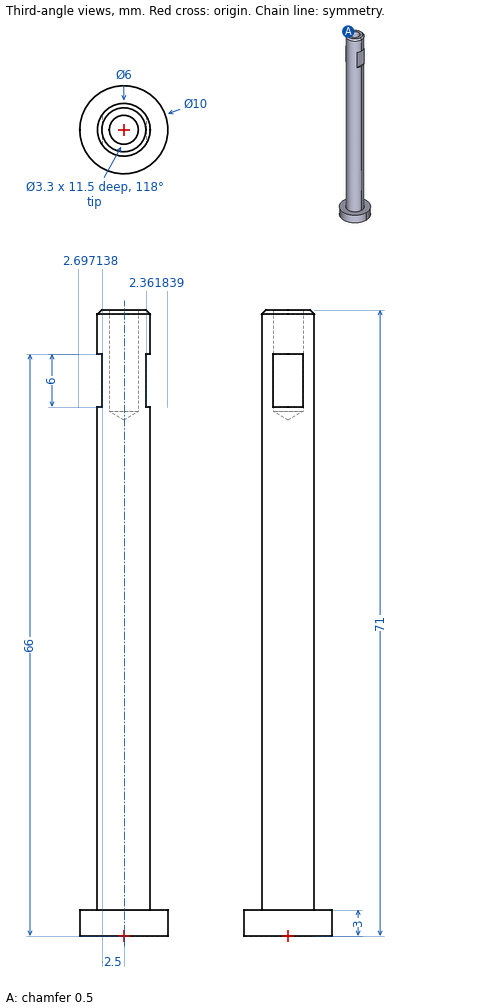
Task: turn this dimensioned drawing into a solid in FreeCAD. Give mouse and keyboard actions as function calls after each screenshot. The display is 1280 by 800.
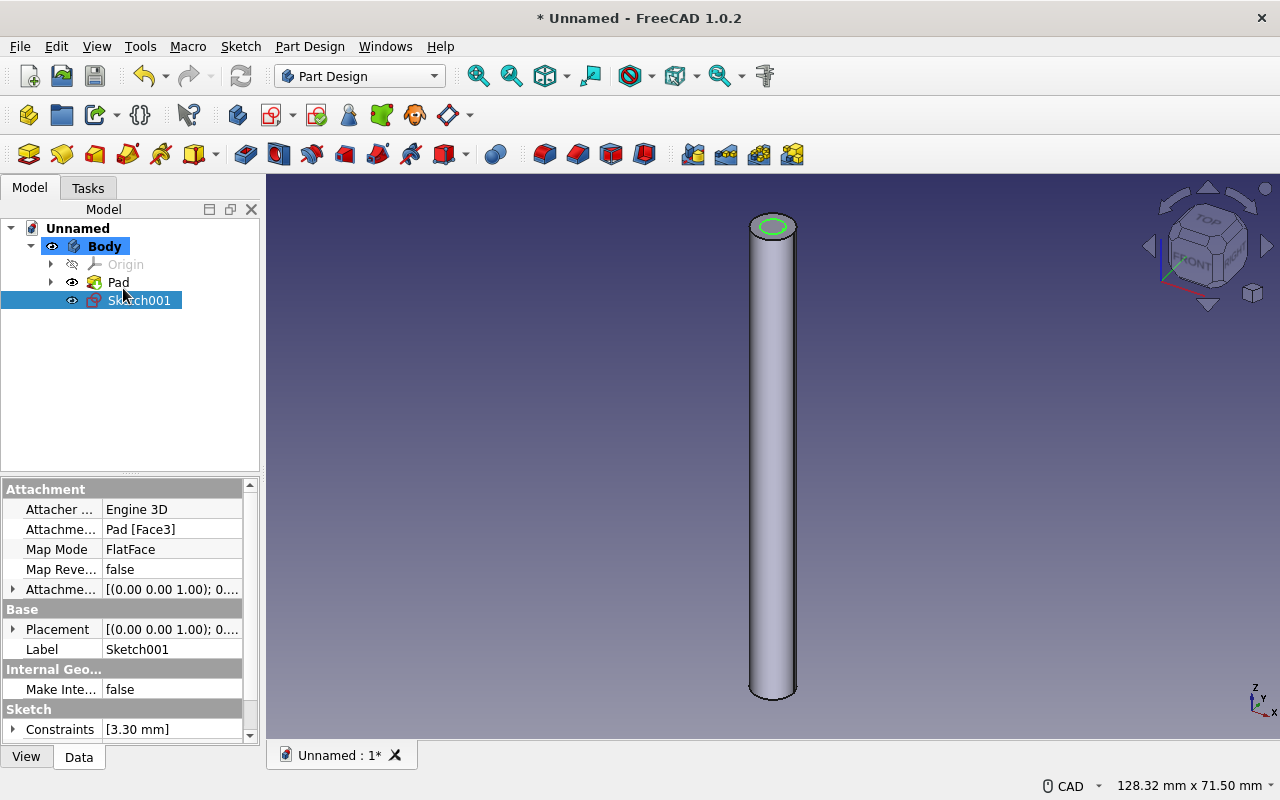
click(279, 154)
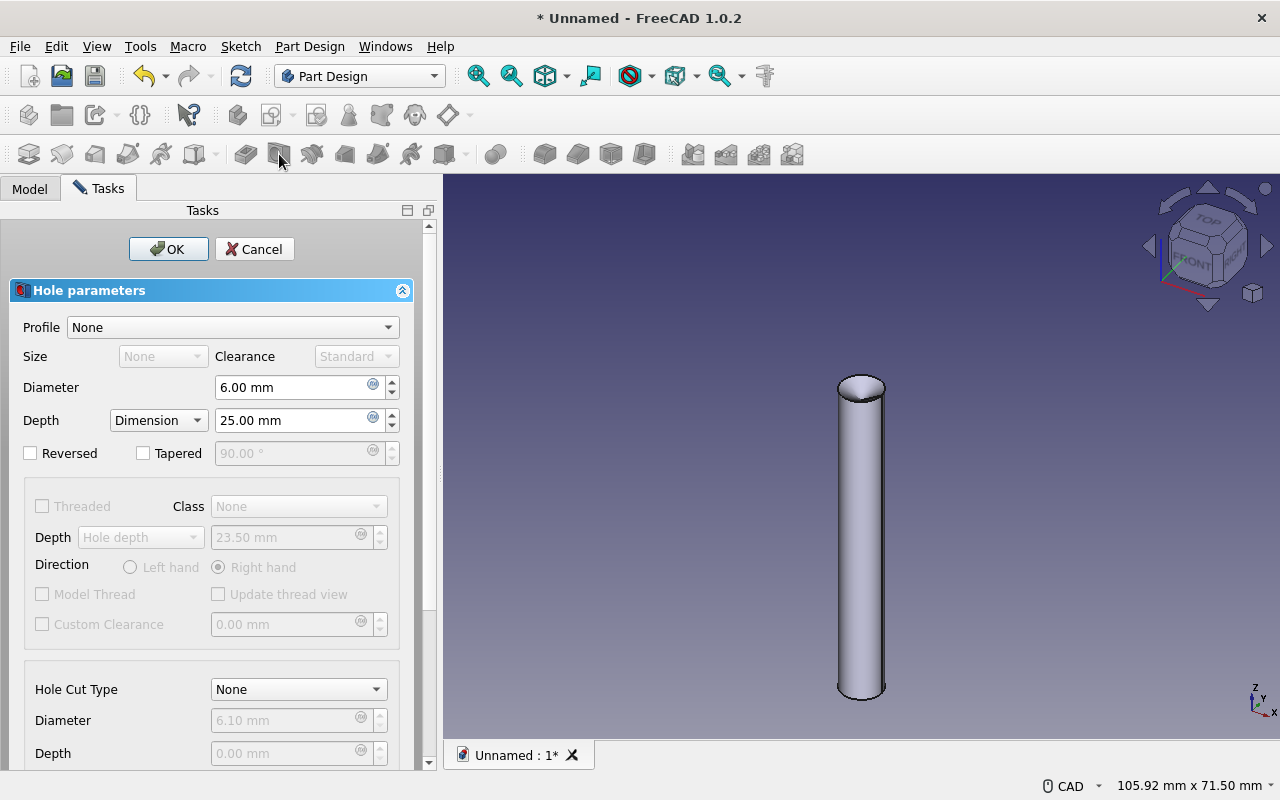
triple_click(300, 388)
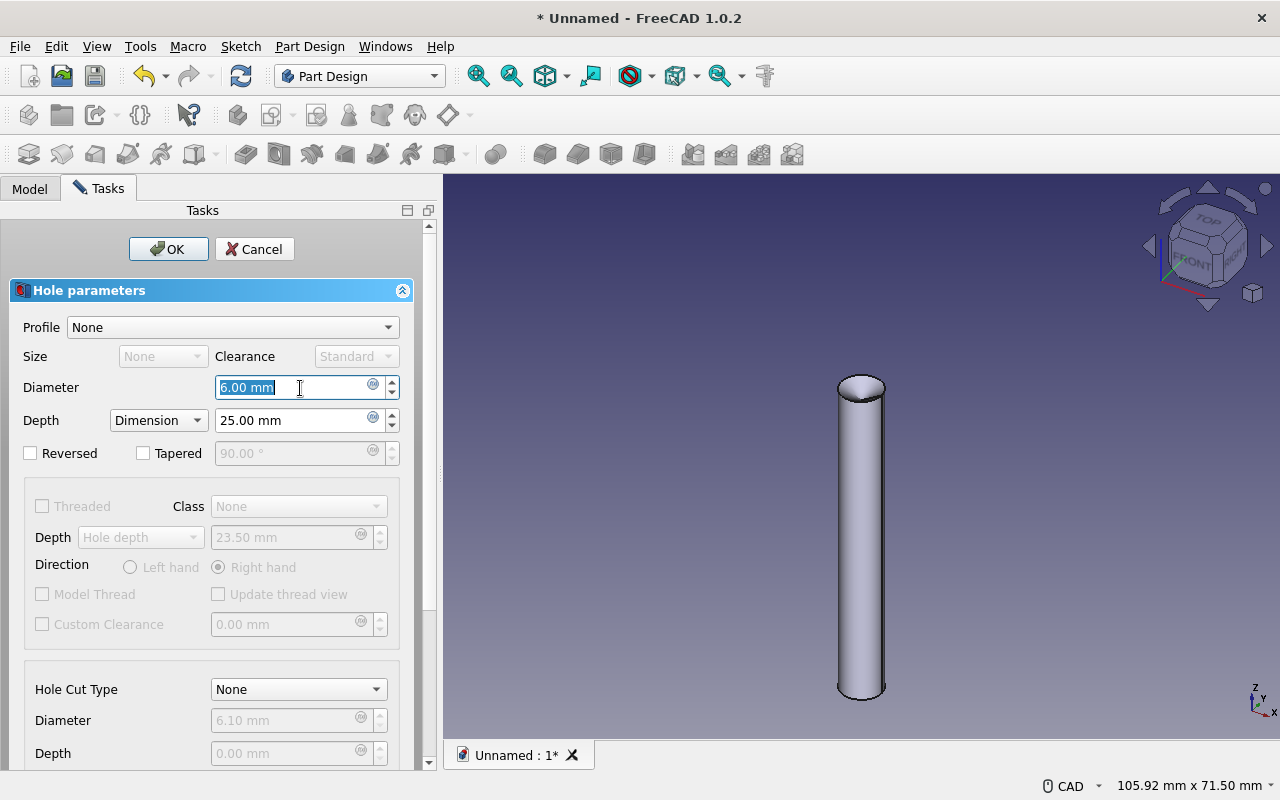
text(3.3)
key(Tab)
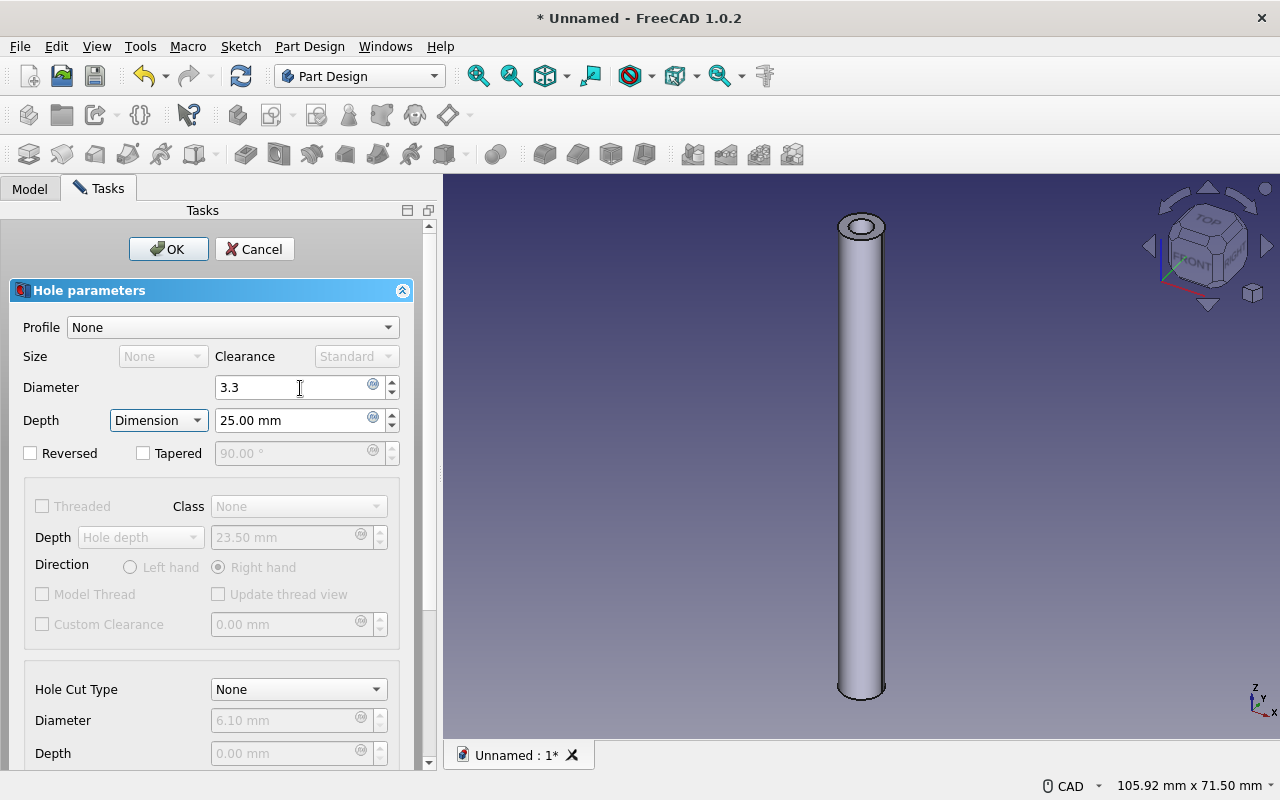
triple_click(300, 420)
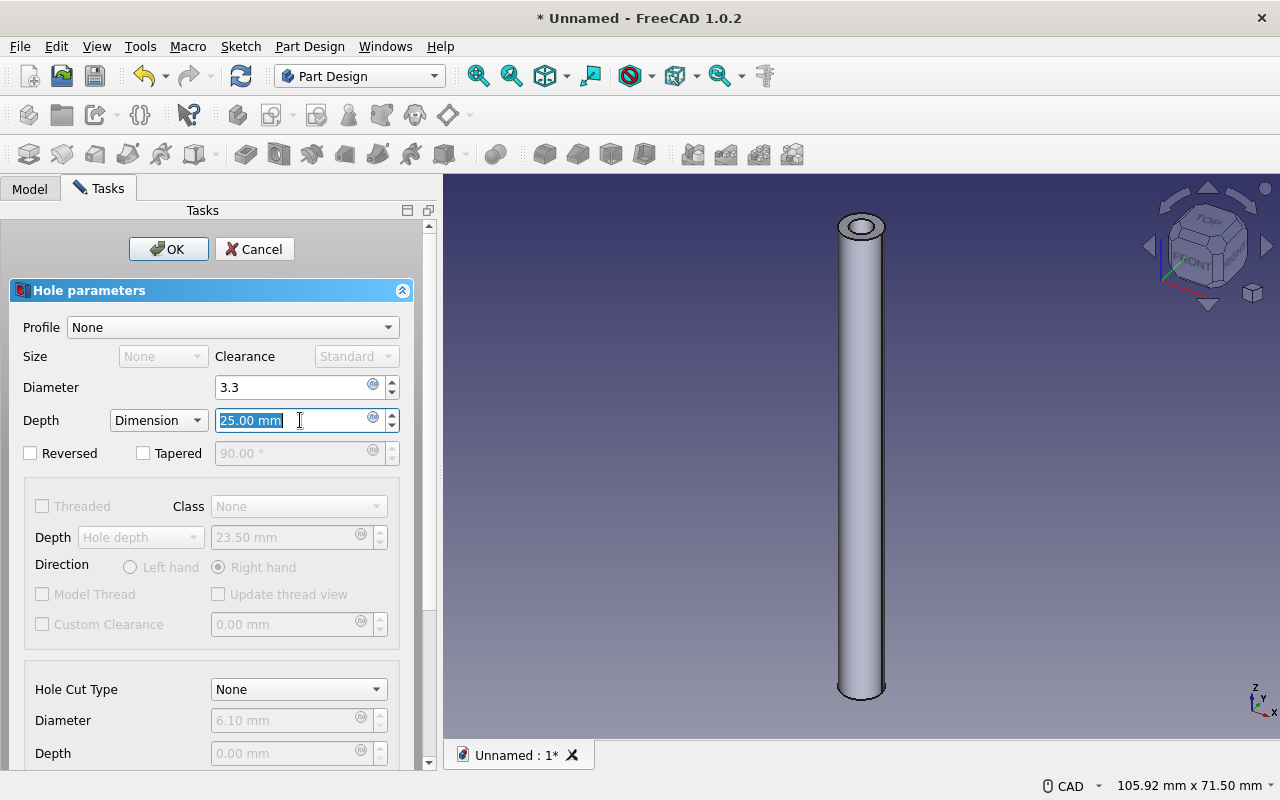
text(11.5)
key(Tab)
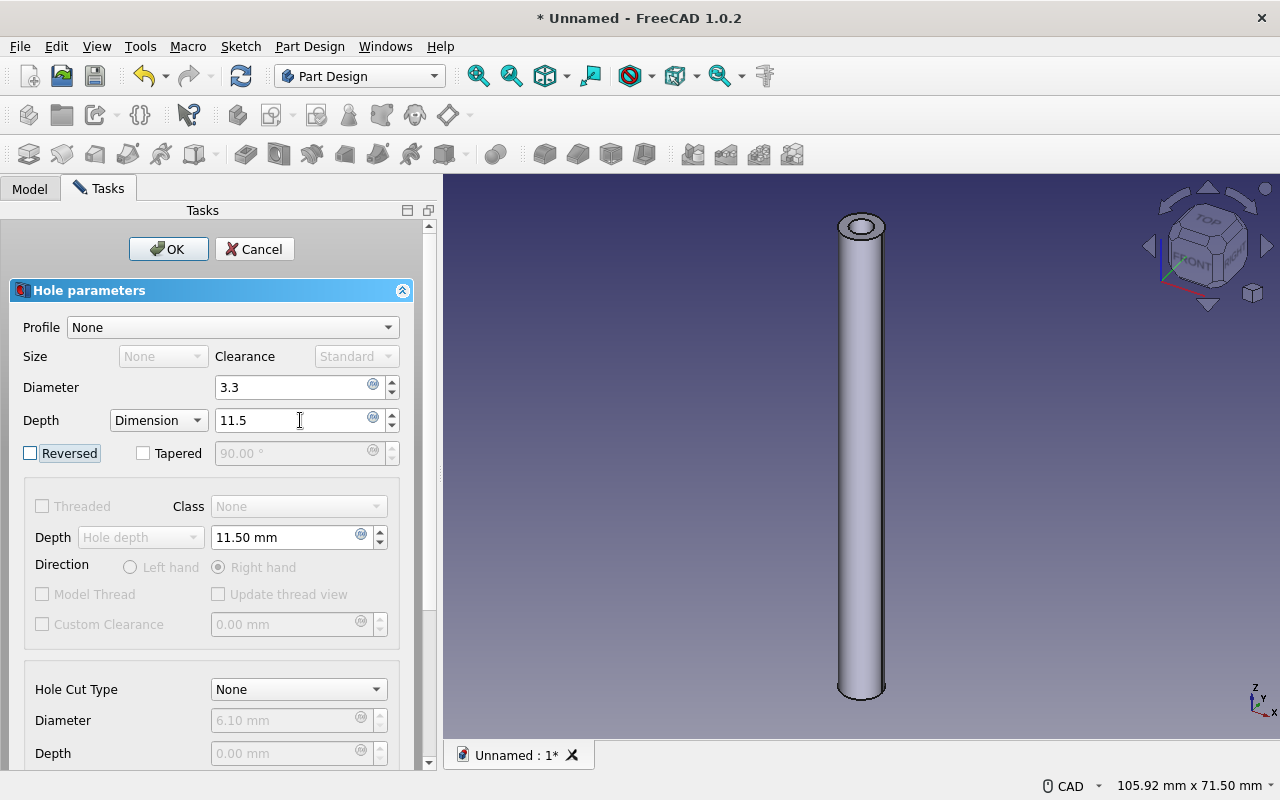
click(169, 249)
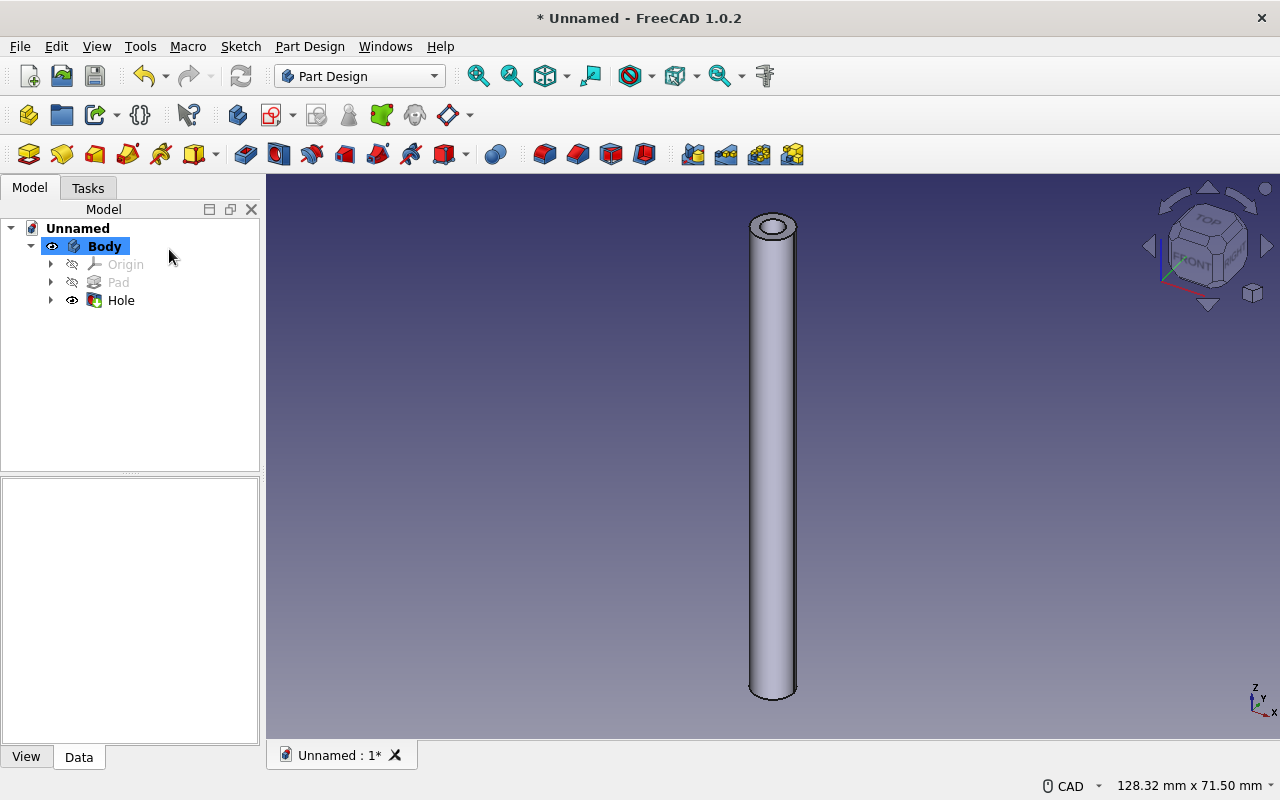
click(752, 219)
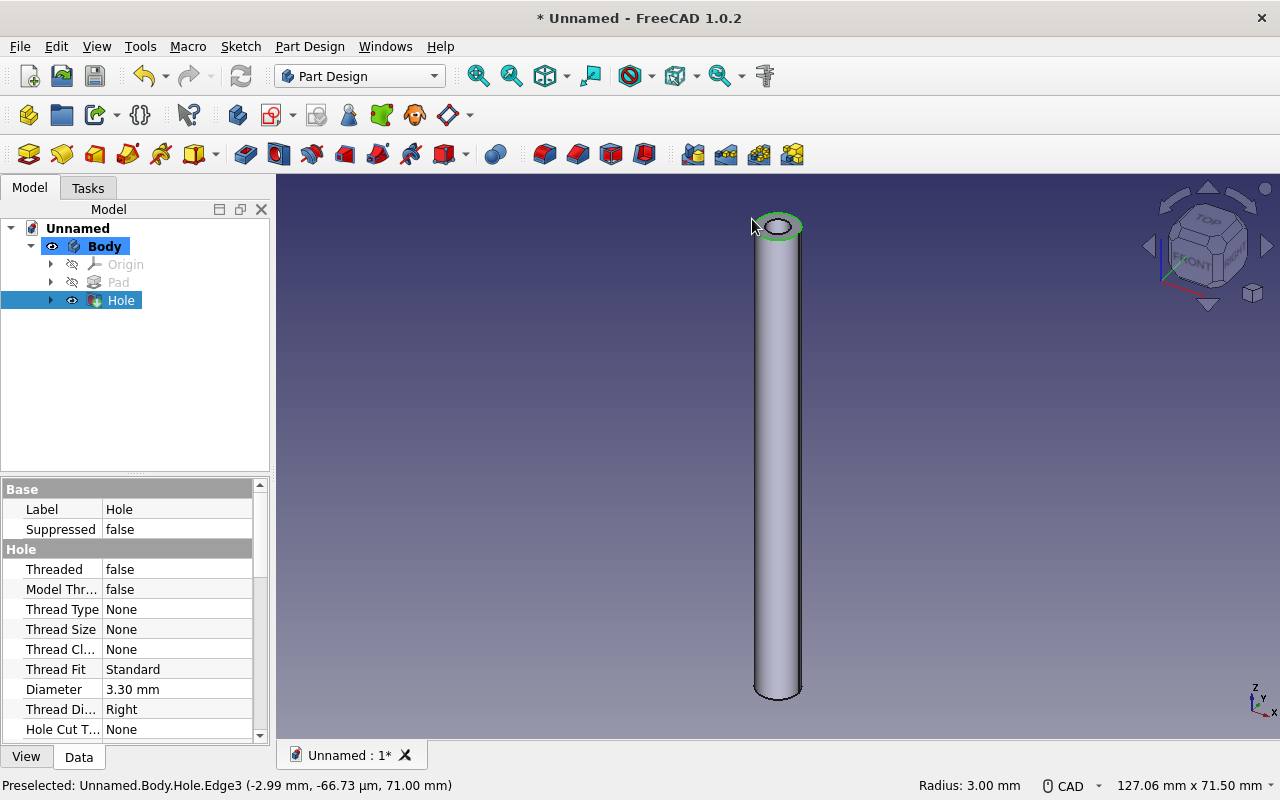
click(578, 154)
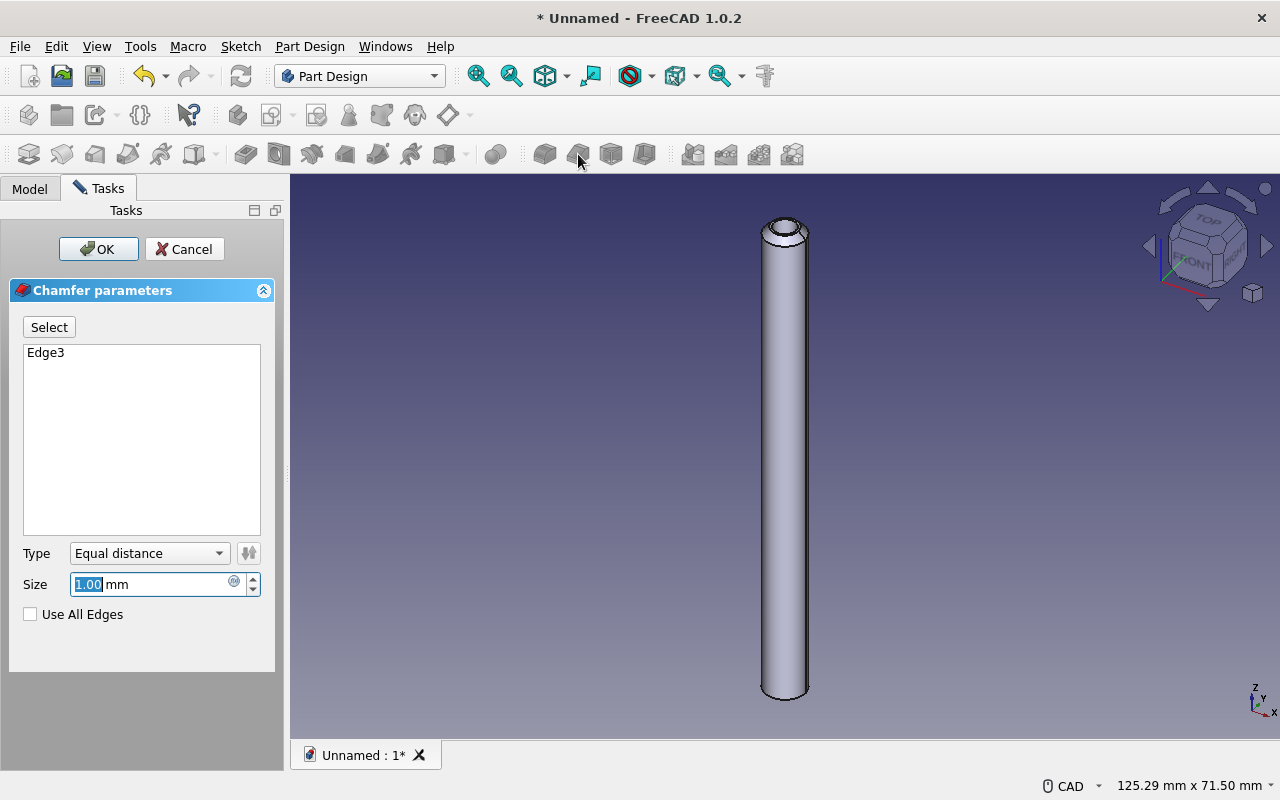
text(0.5)
key(Tab)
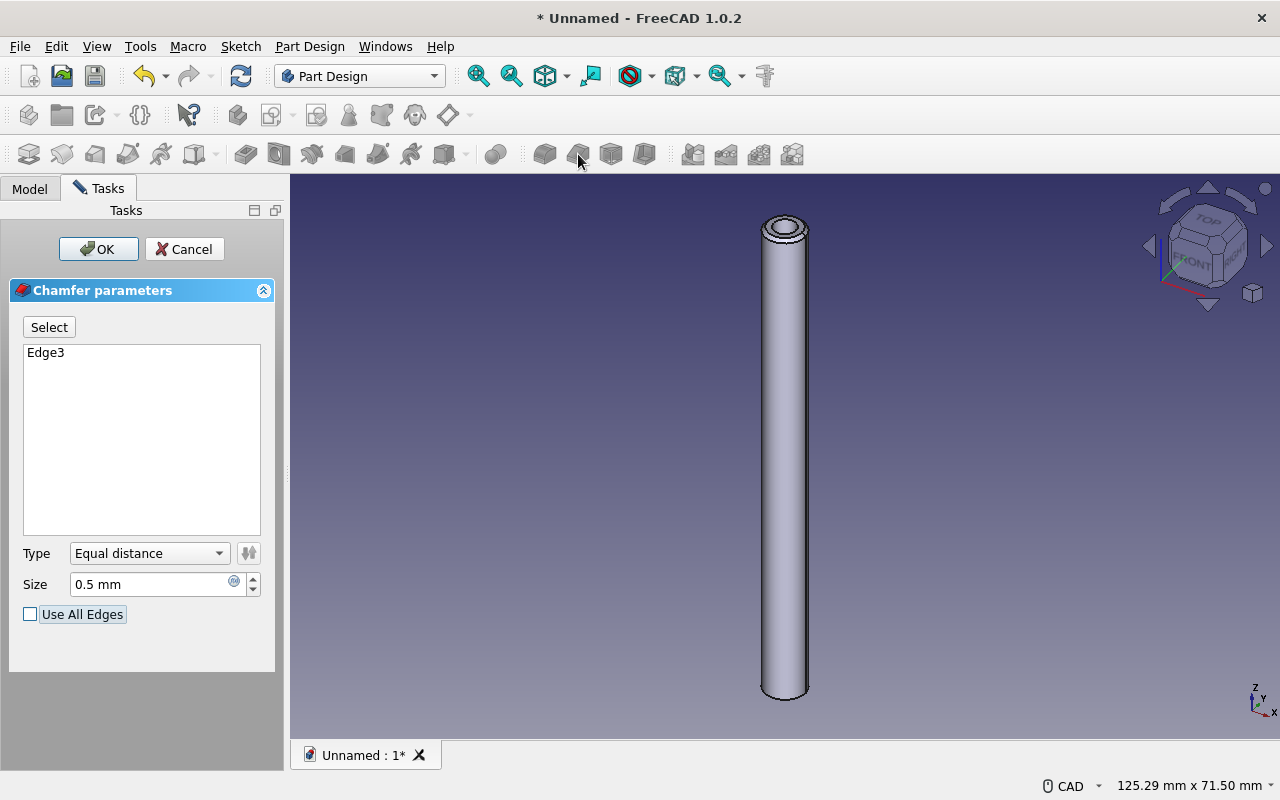
click(99, 249)